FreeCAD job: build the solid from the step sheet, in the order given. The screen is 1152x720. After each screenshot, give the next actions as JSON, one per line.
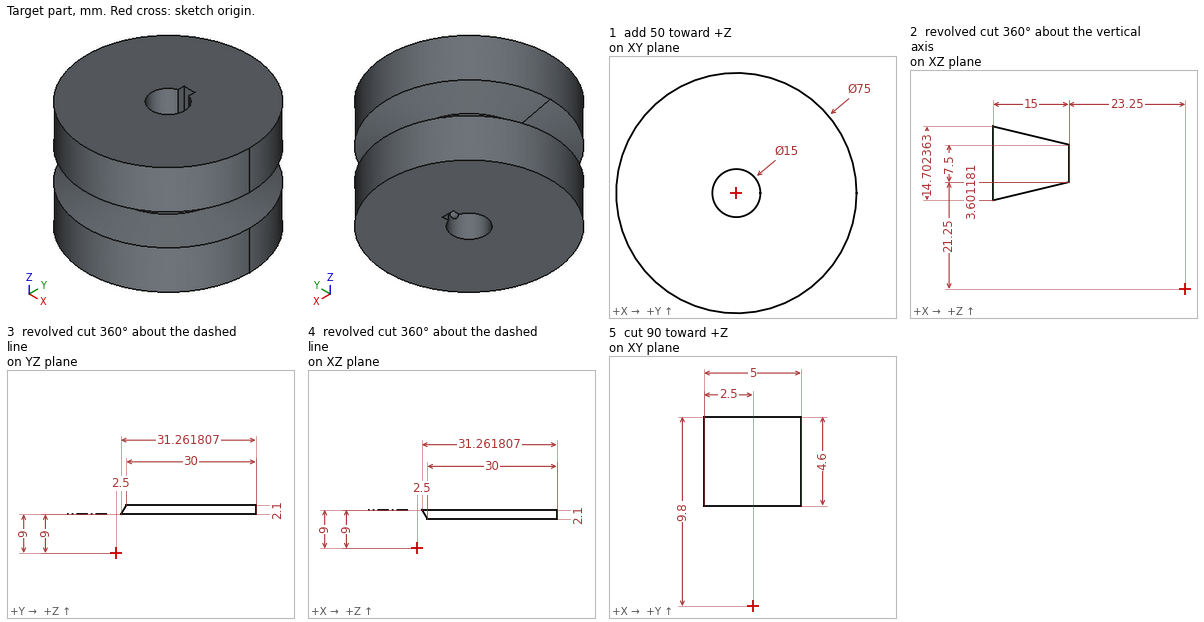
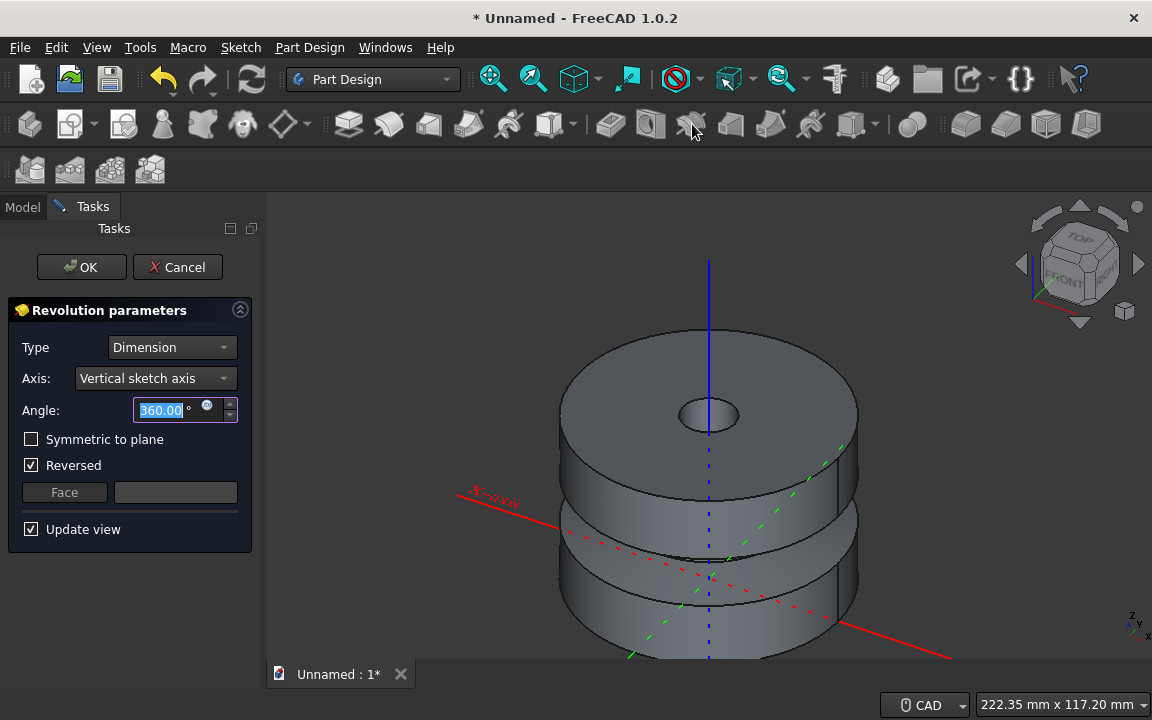
{"action": "left_click", "coordinate": [82, 267]}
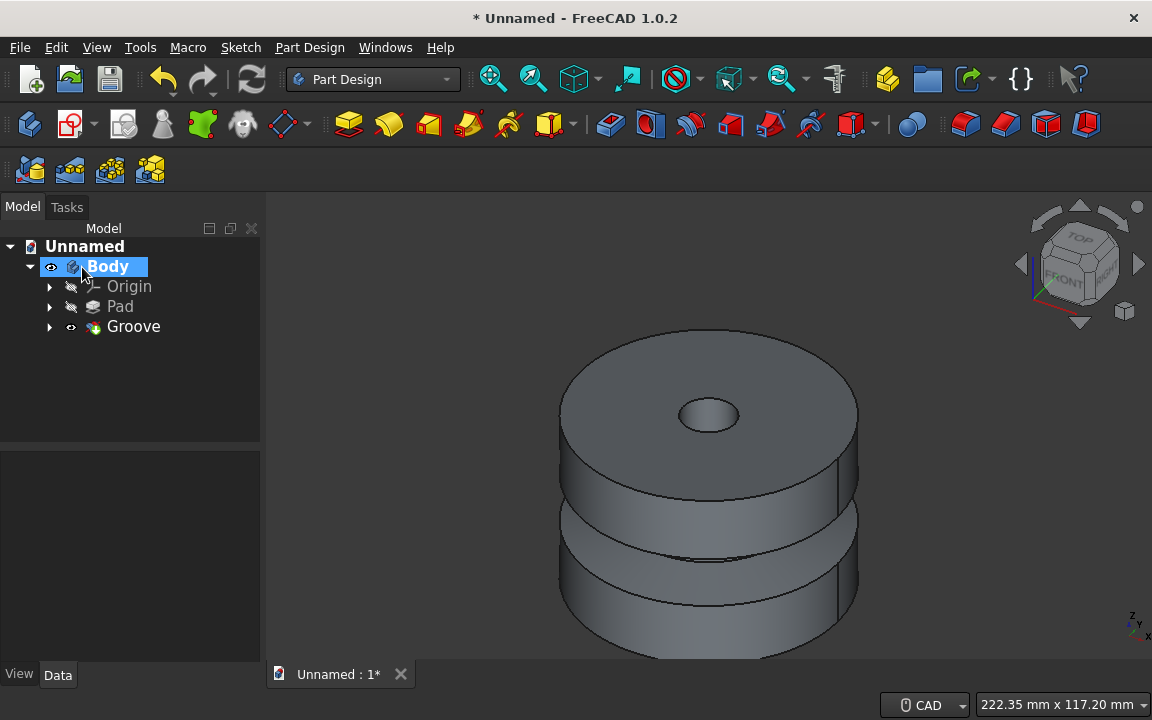
{"action": "left_click", "coordinate": [494, 80]}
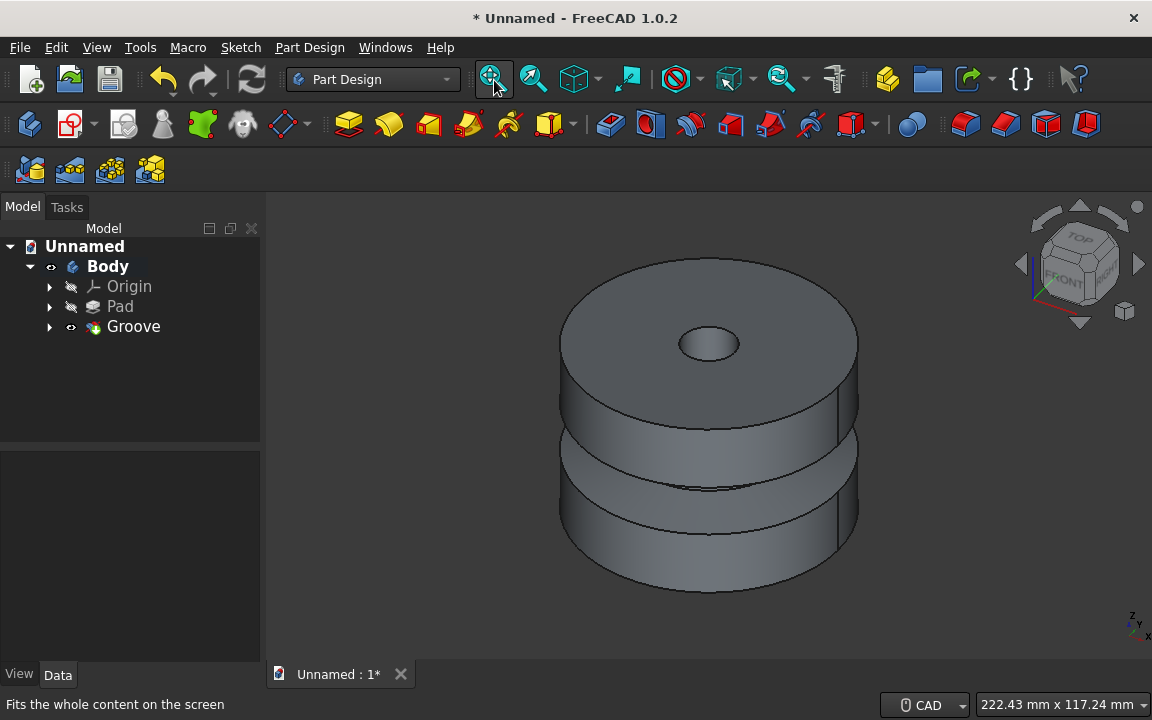
{"action": "left_click", "coordinate": [70, 124]}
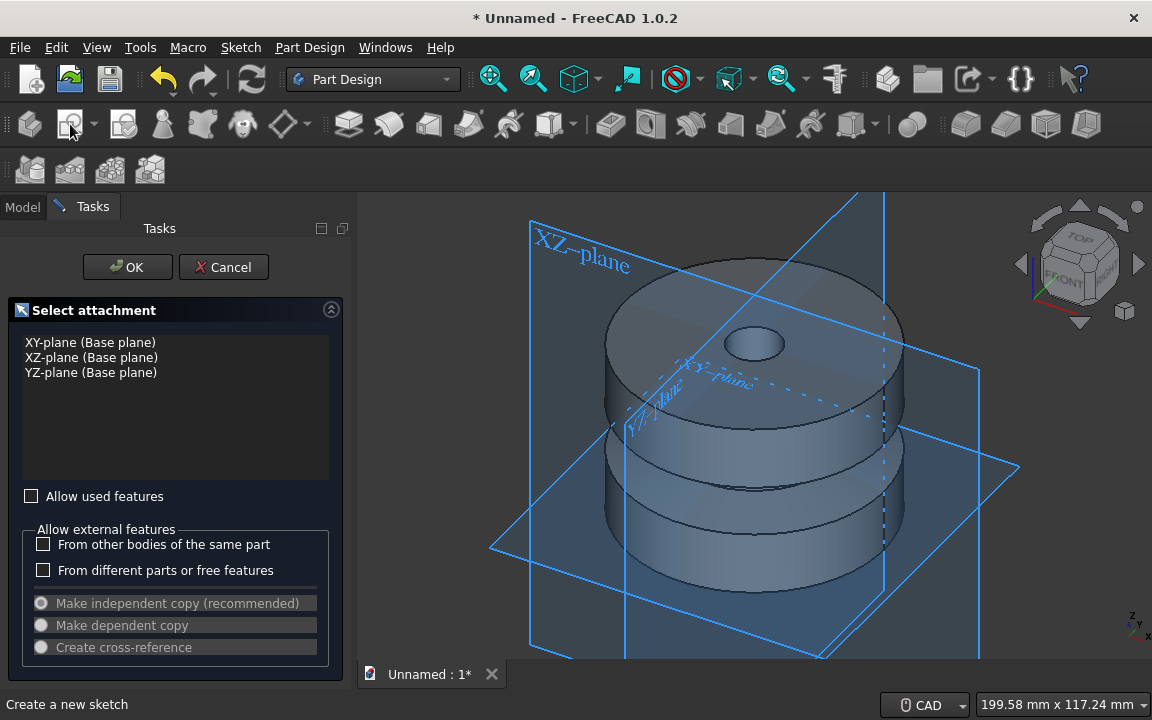
{"action": "left_click", "coordinate": [82, 372]}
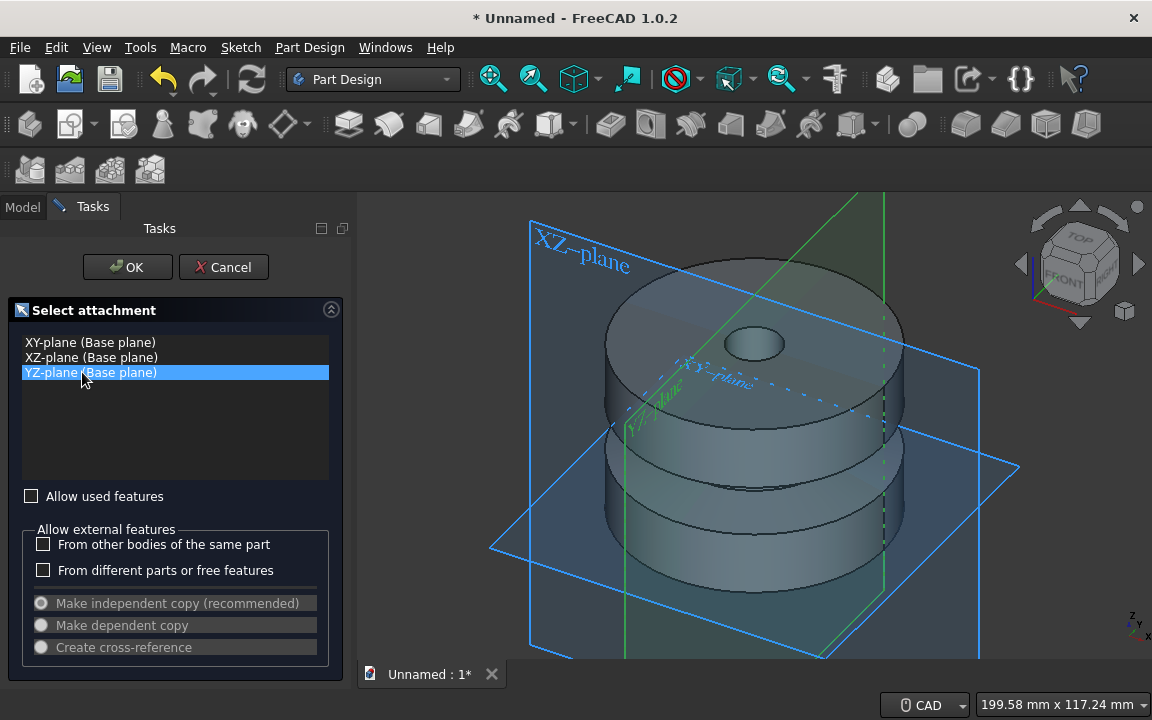
{"action": "left_click", "coordinate": [128, 267]}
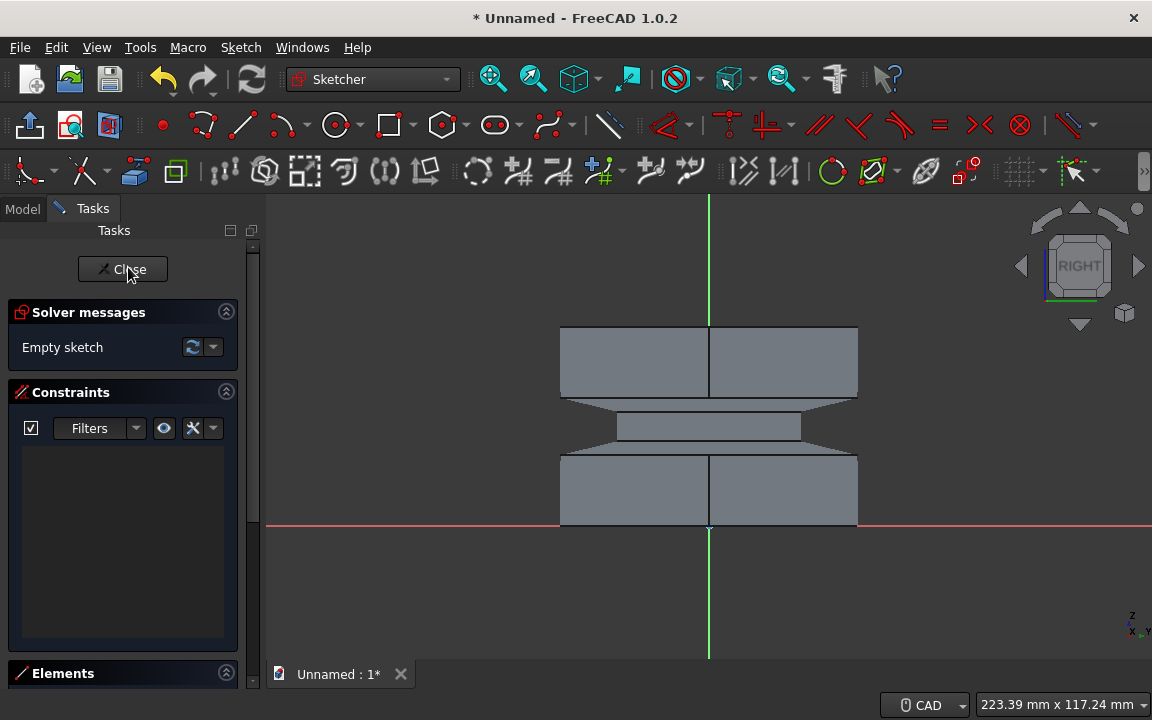
{"action": "key", "text": "q s"}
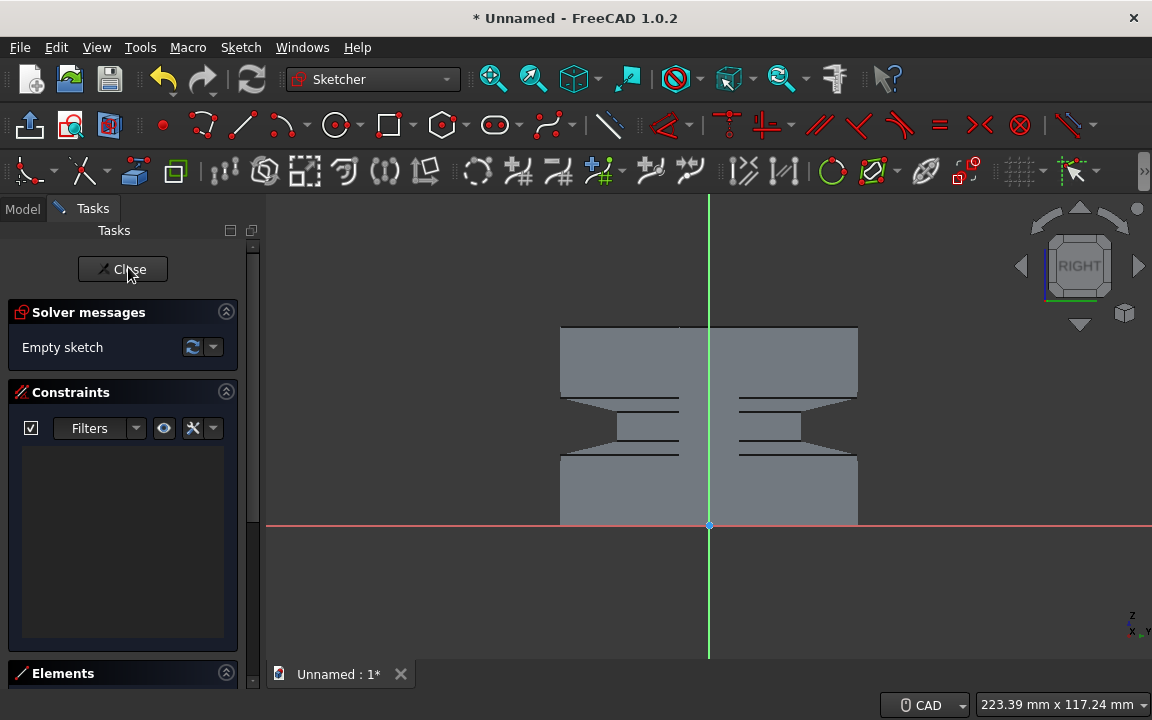
{"action": "scroll", "coordinate": [815, 549], "scroll_direction": "up", "scroll_amount": 5}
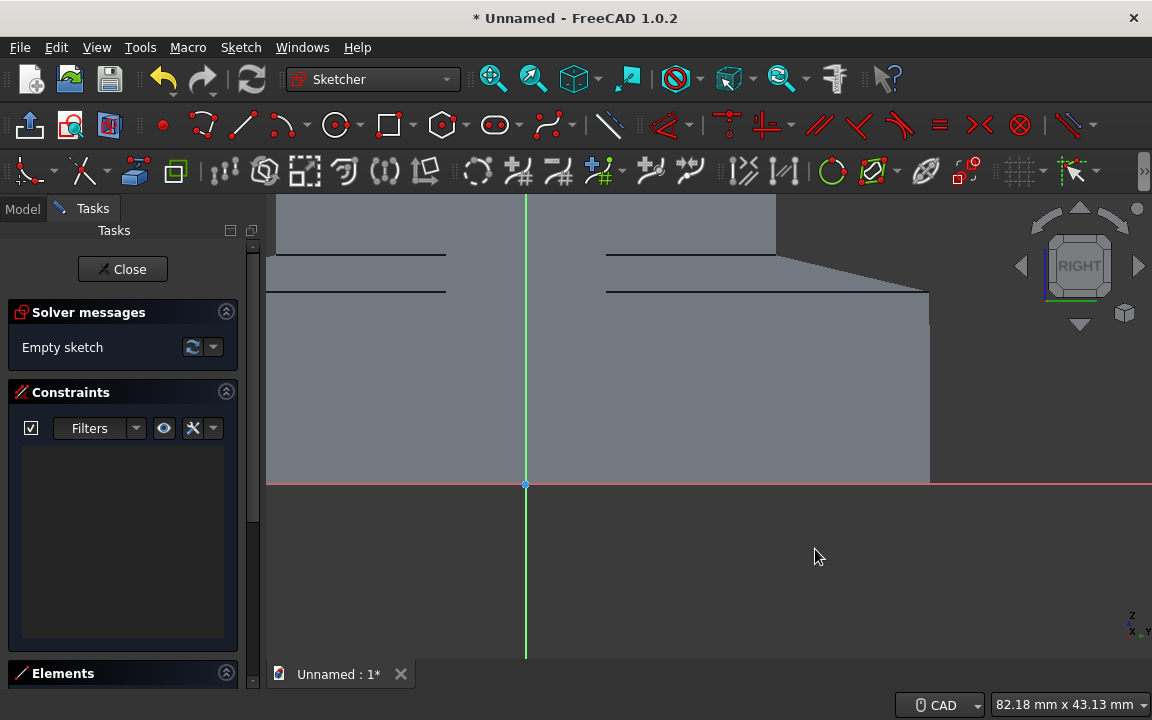
{"action": "left_click", "coordinate": [204, 126]}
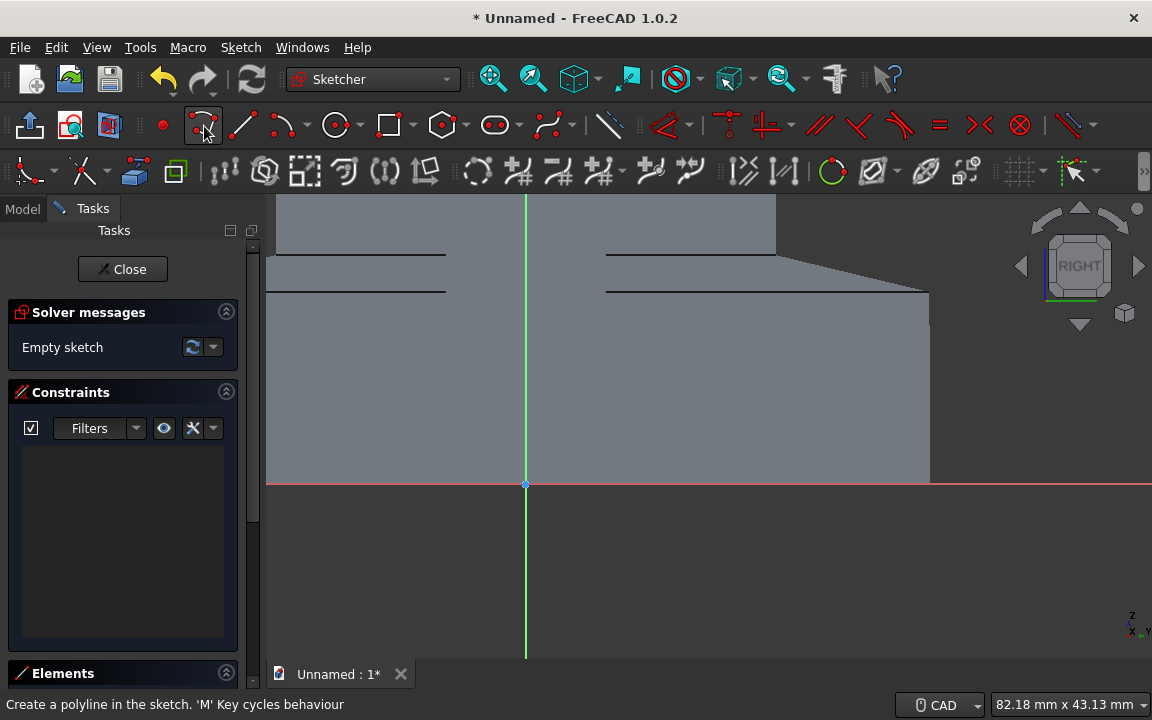
{"action": "left_click", "coordinate": [539, 387]}
{"action": "left_click", "coordinate": [876, 387]}
{"action": "left_click", "coordinate": [876, 365]}
{"action": "left_click", "coordinate": [553, 365]}
{"action": "left_click", "coordinate": [539, 388]}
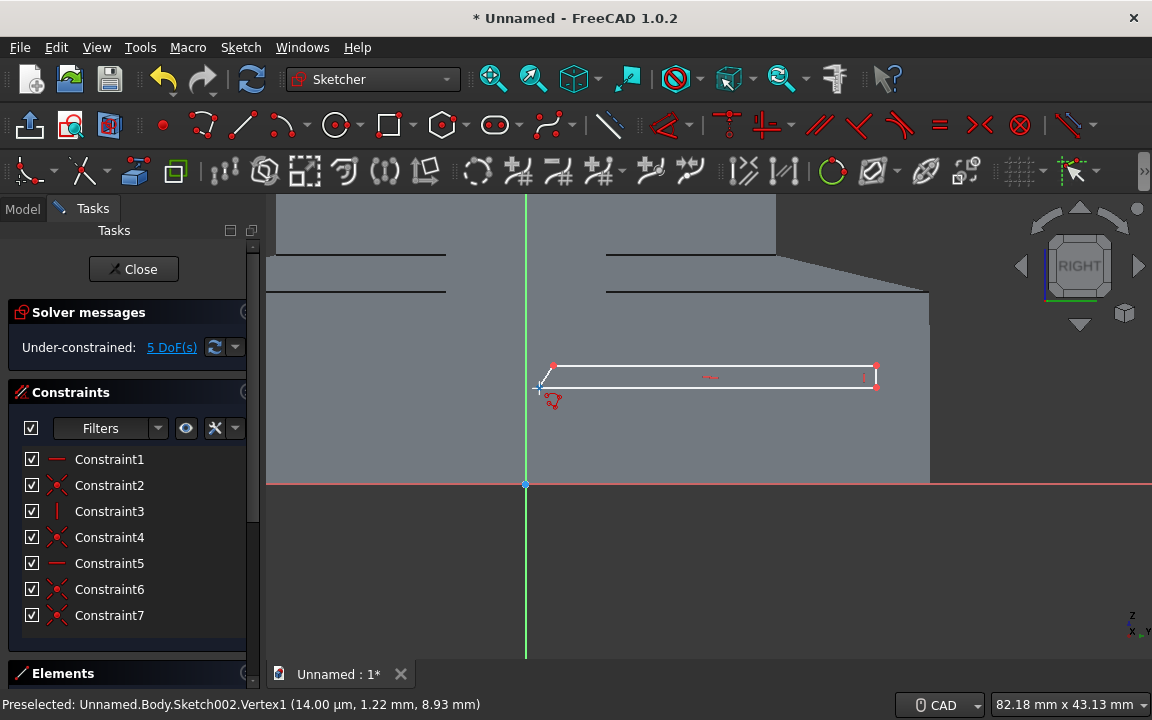
{"action": "left_click", "coordinate": [244, 126]}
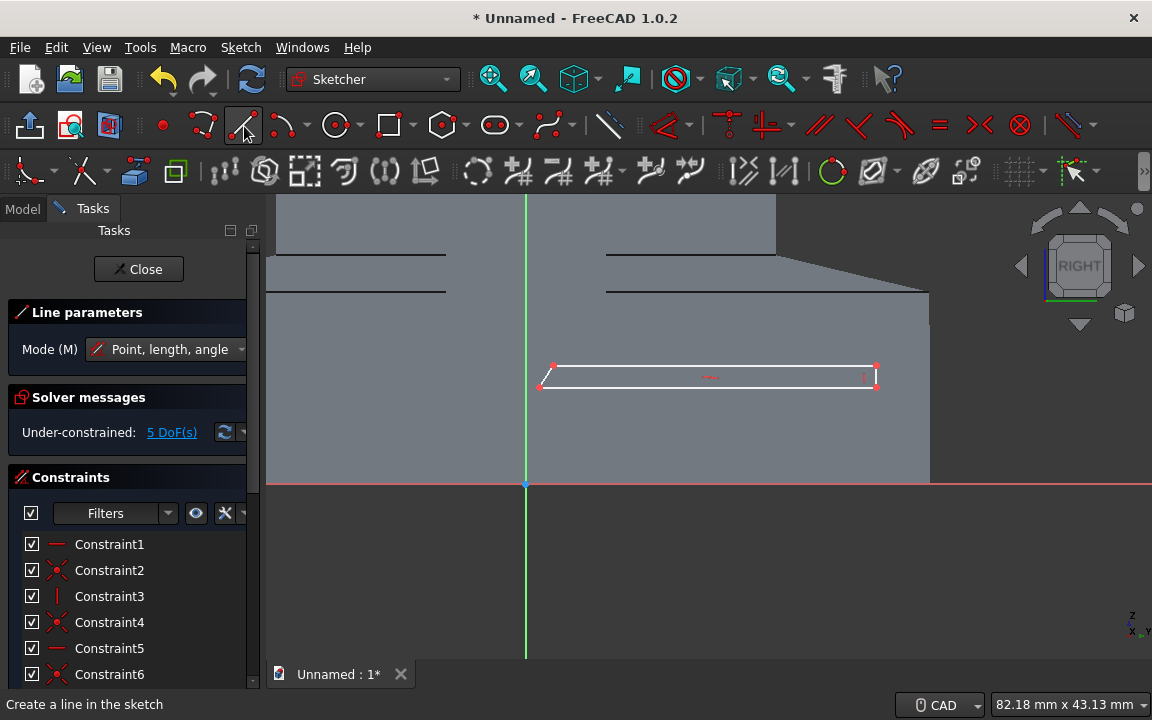
{"action": "left_click", "coordinate": [505, 387]}
{"action": "left_click", "coordinate": [404, 387]}
{"action": "key", "text": "Escape"}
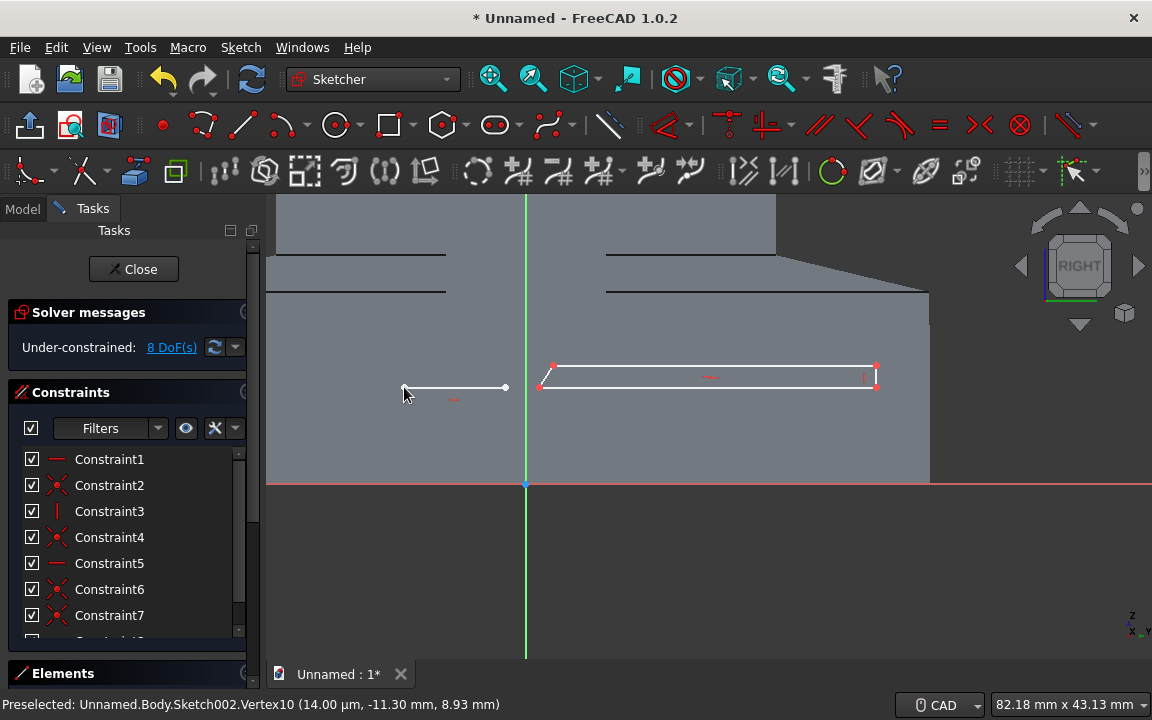
{"action": "left_click", "coordinate": [475, 388]}